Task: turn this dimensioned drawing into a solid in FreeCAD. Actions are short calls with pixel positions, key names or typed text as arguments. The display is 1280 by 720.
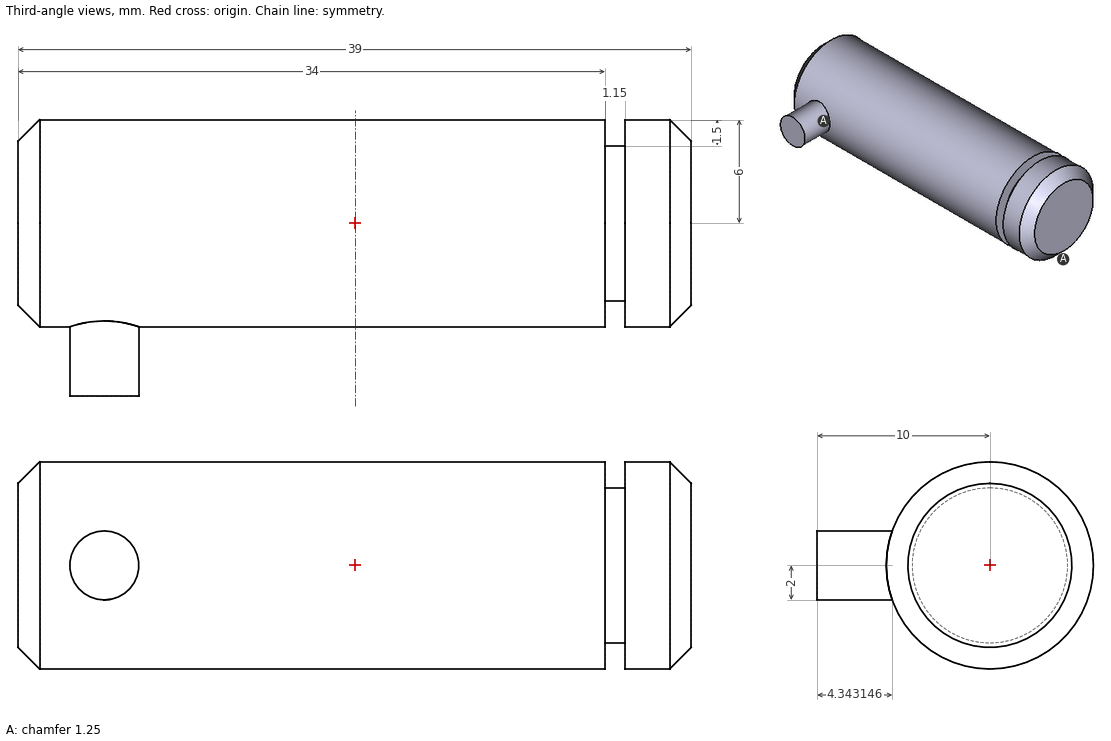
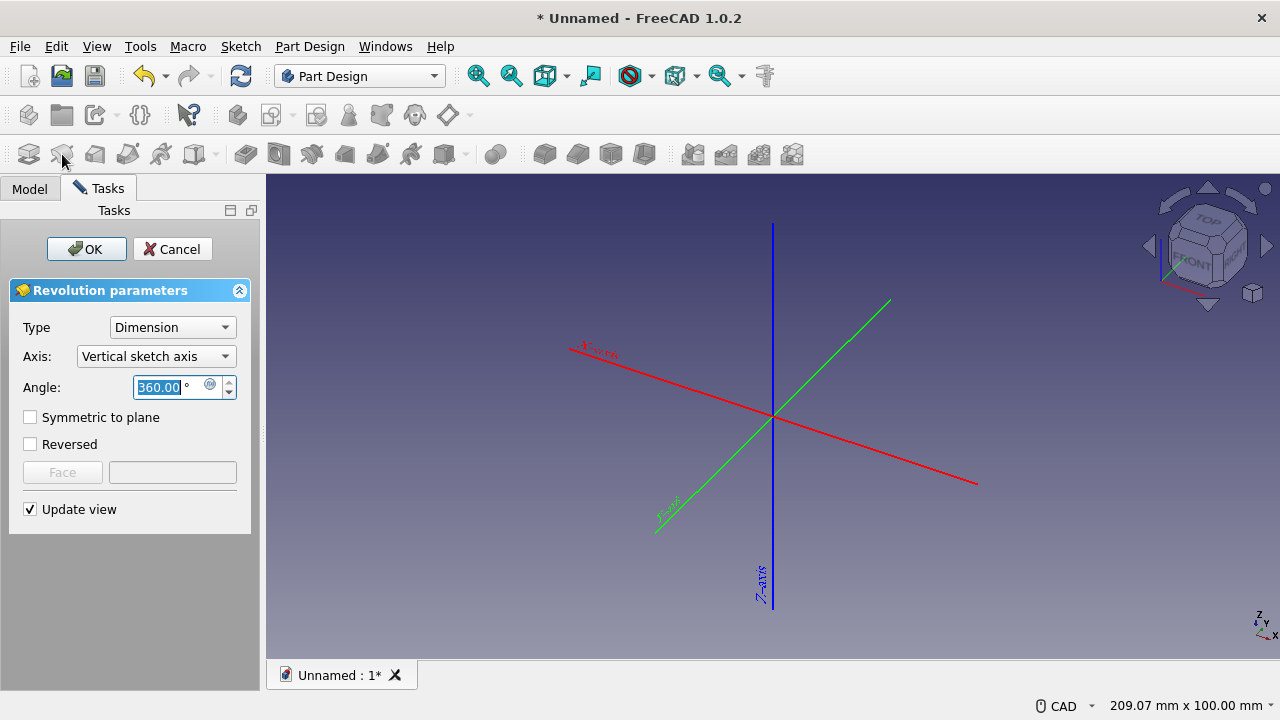
click(157, 356)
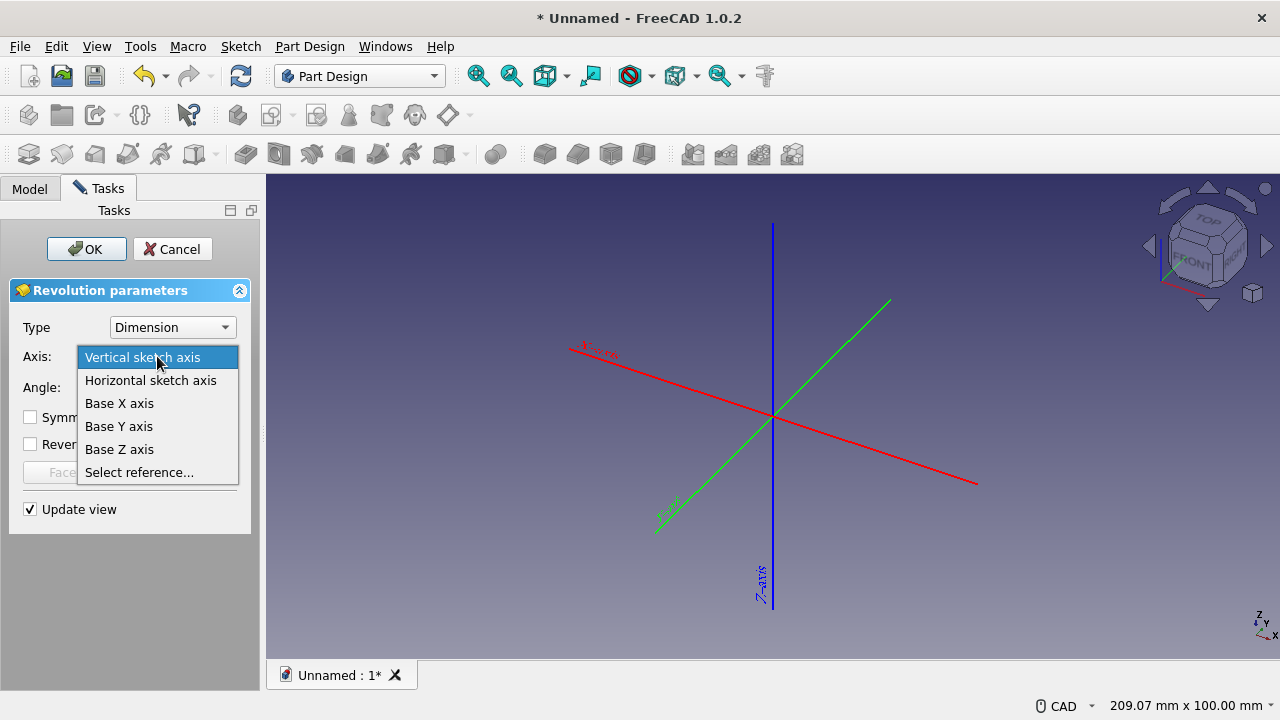
click(156, 380)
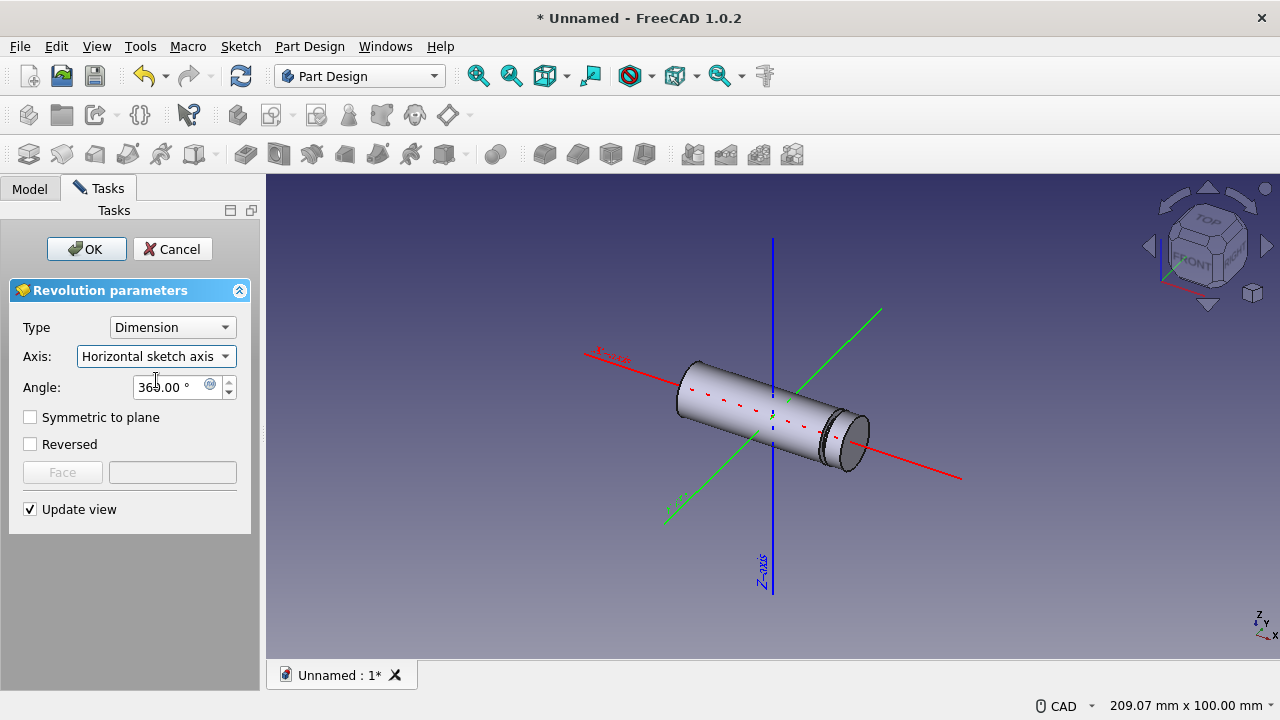
click(87, 249)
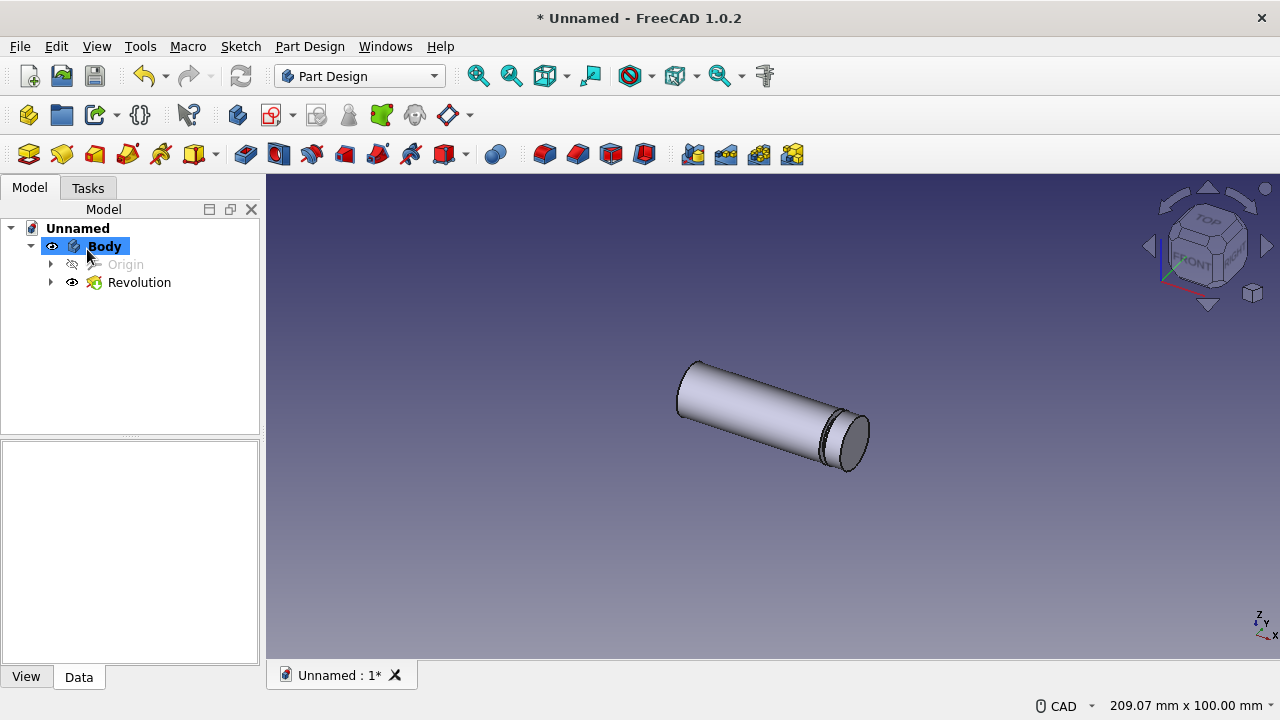
key(v)
key(f)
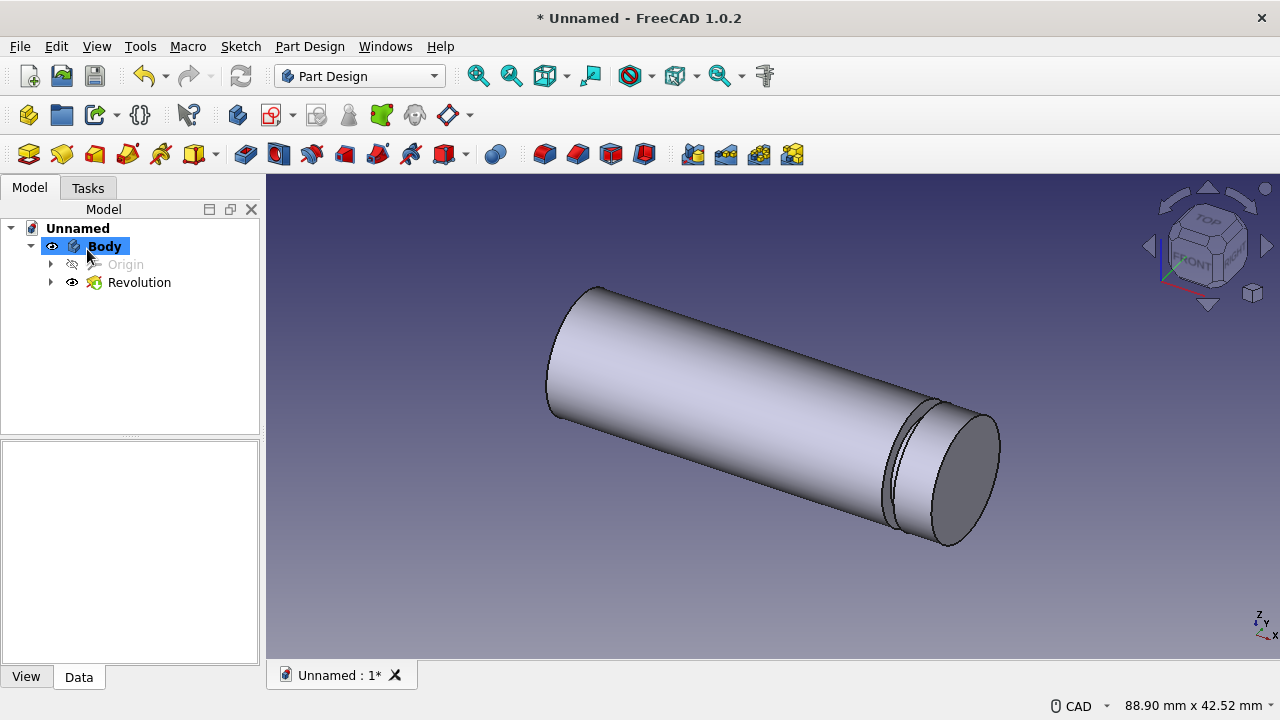
click(51, 264)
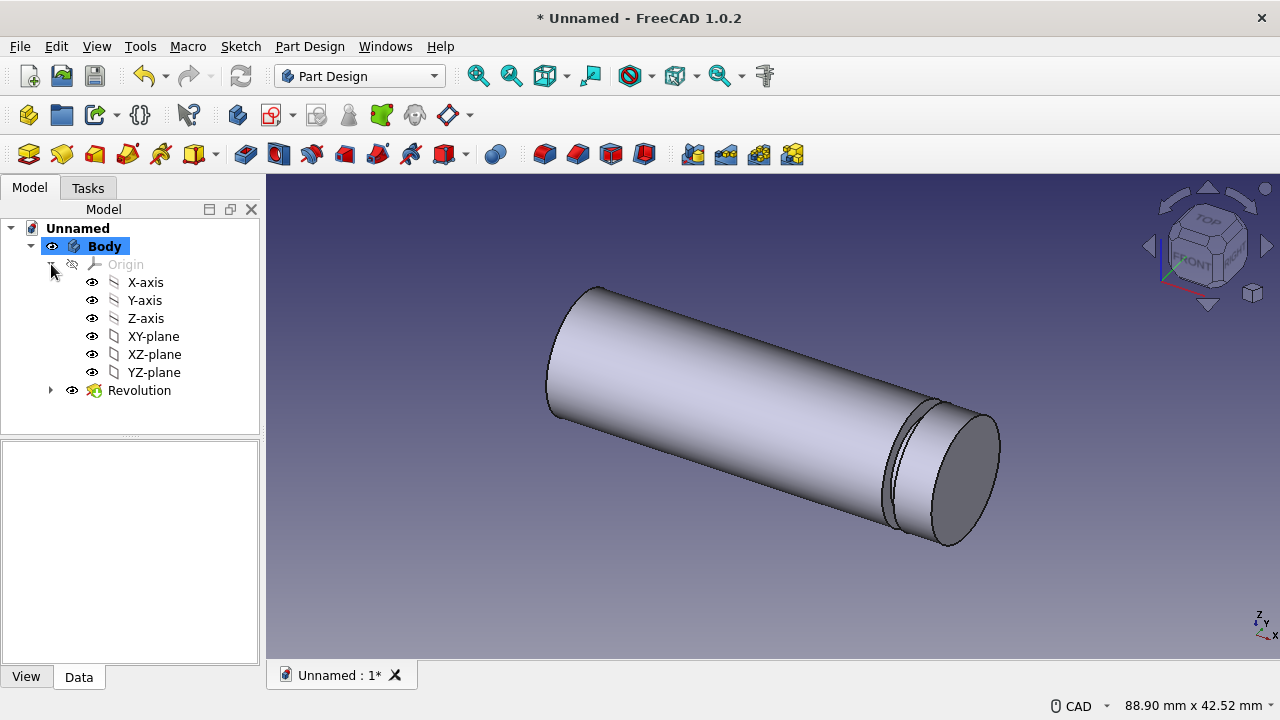
click(137, 372)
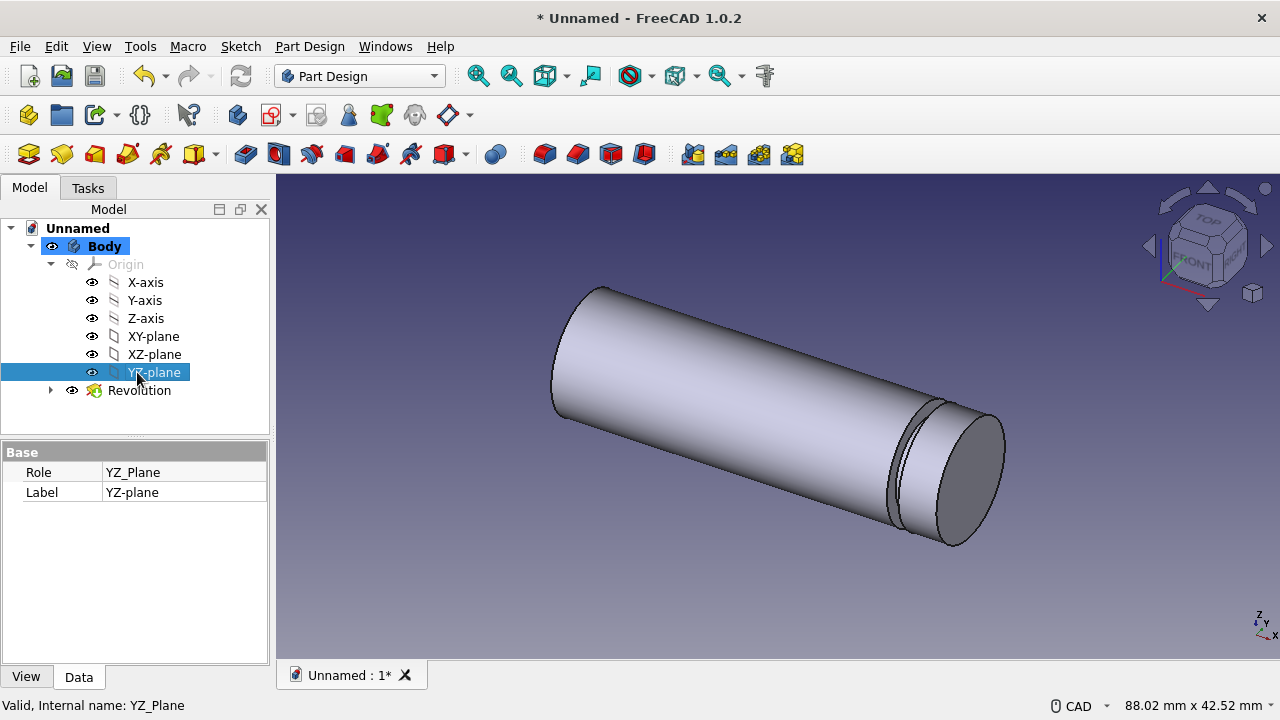
click(448, 116)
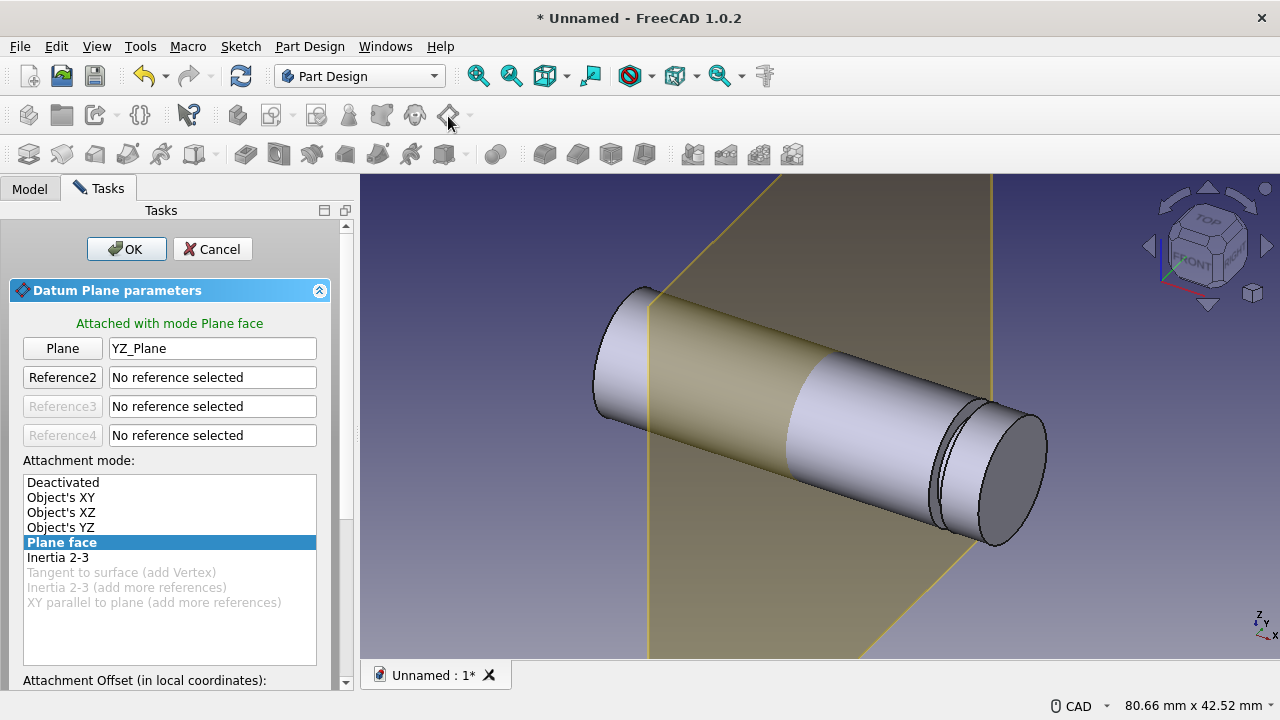
scroll(346, 455, down, 3)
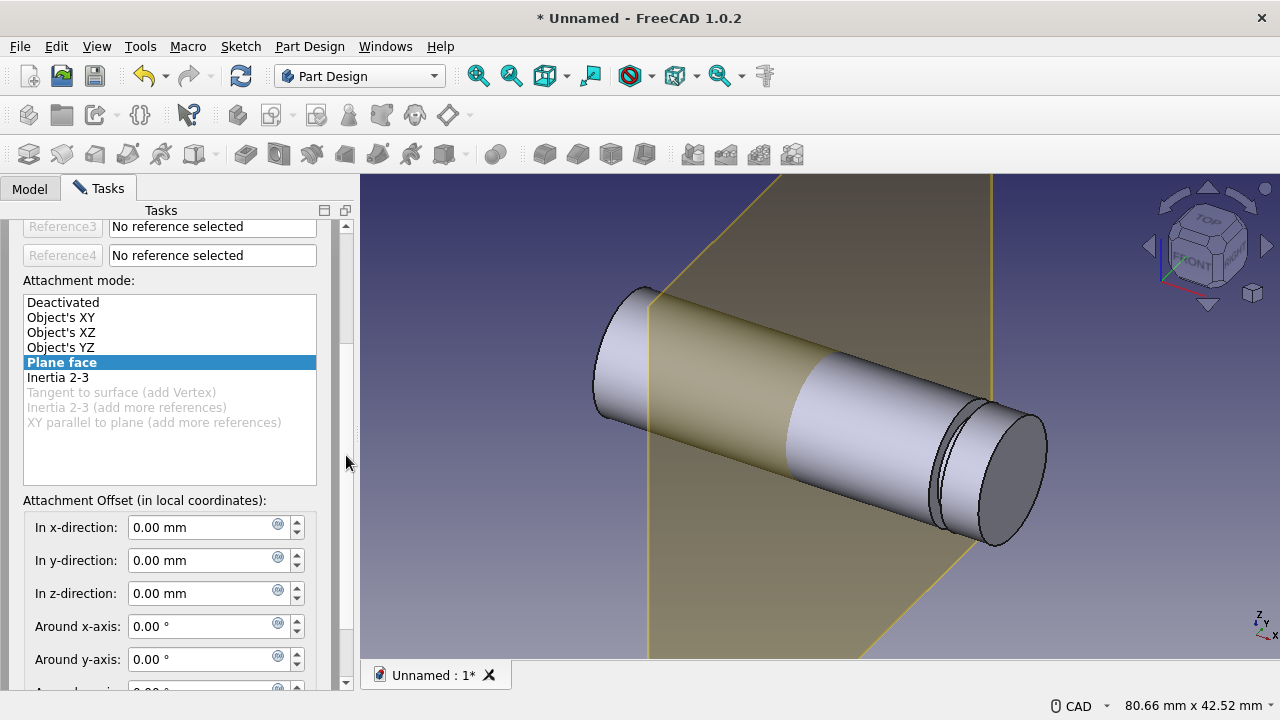
triple_click(210, 594)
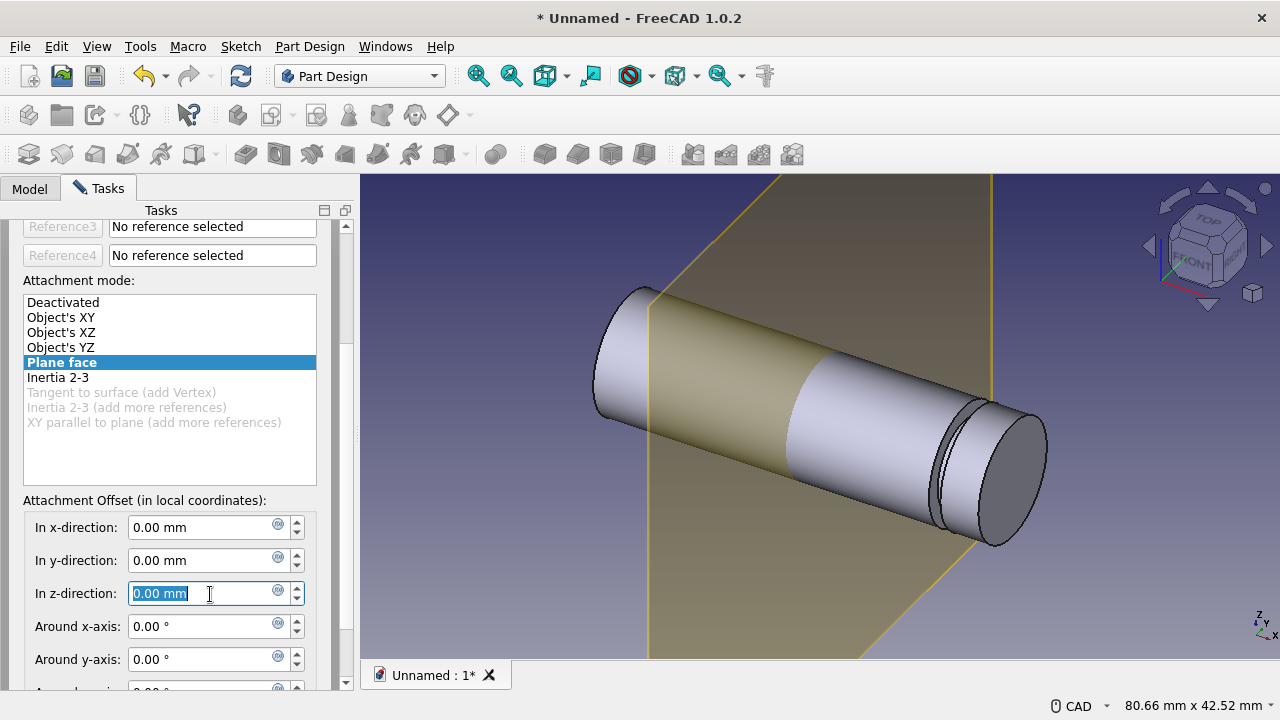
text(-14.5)
key(Tab)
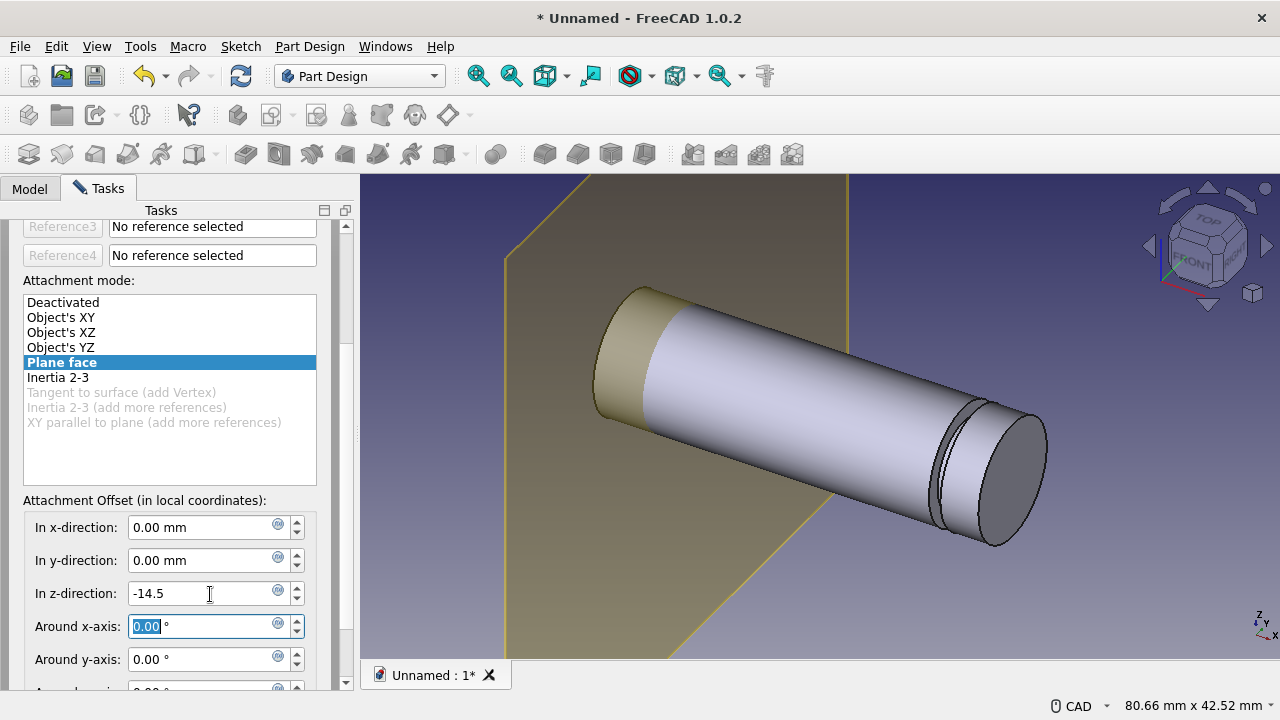
scroll(346, 455, up, 4)